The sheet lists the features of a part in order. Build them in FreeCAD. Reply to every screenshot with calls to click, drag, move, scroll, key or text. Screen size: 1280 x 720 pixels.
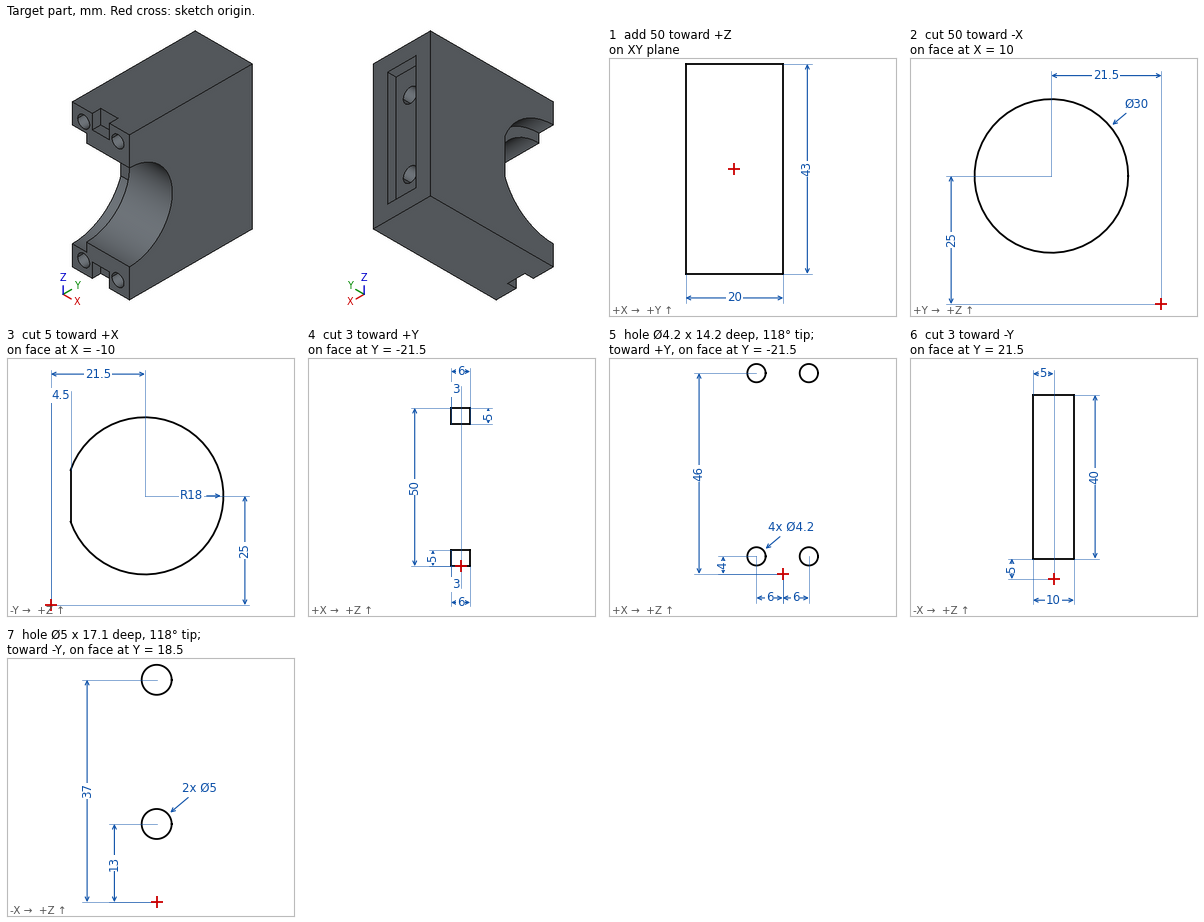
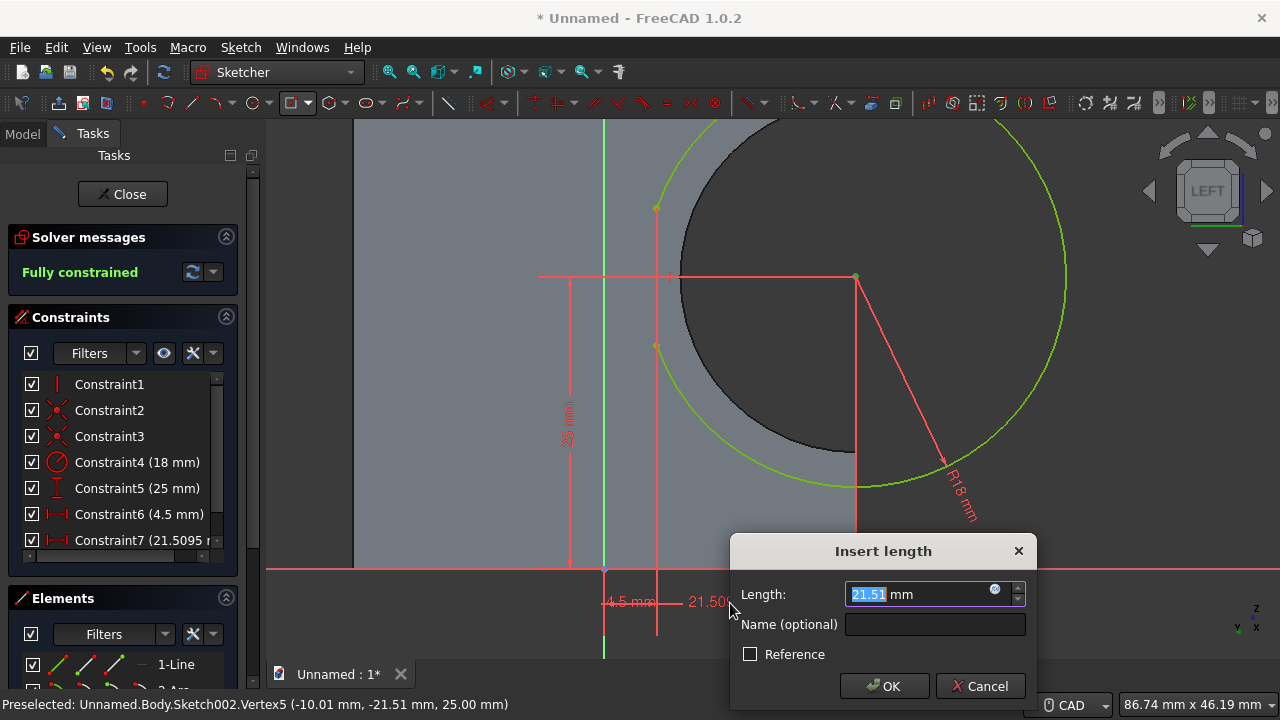
text(21.5)
key(Return)
key(Escape)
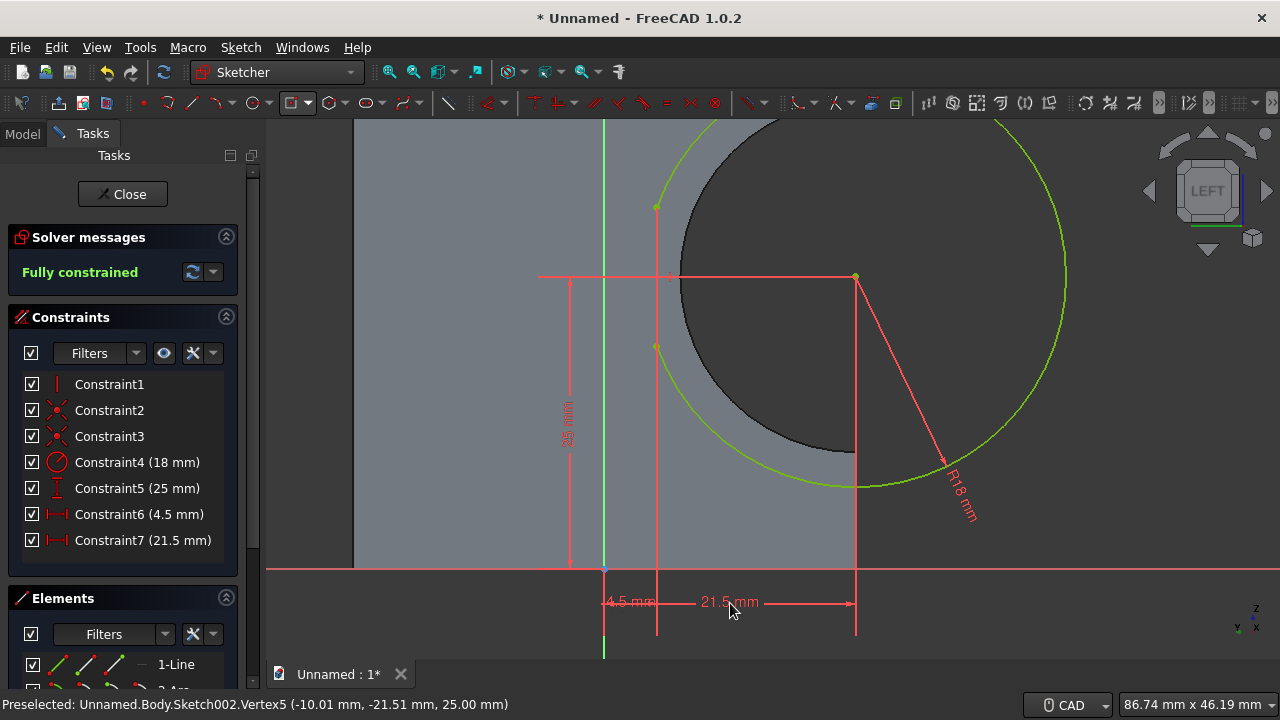
click(123, 194)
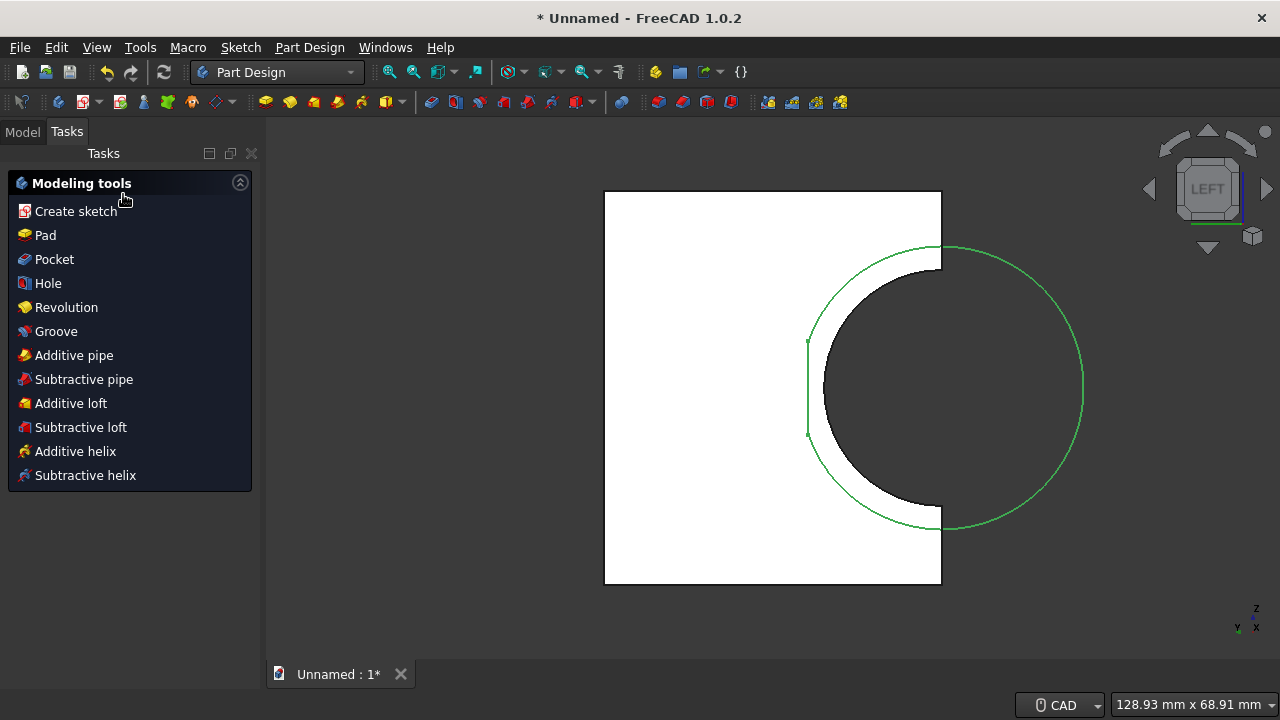
click(432, 102)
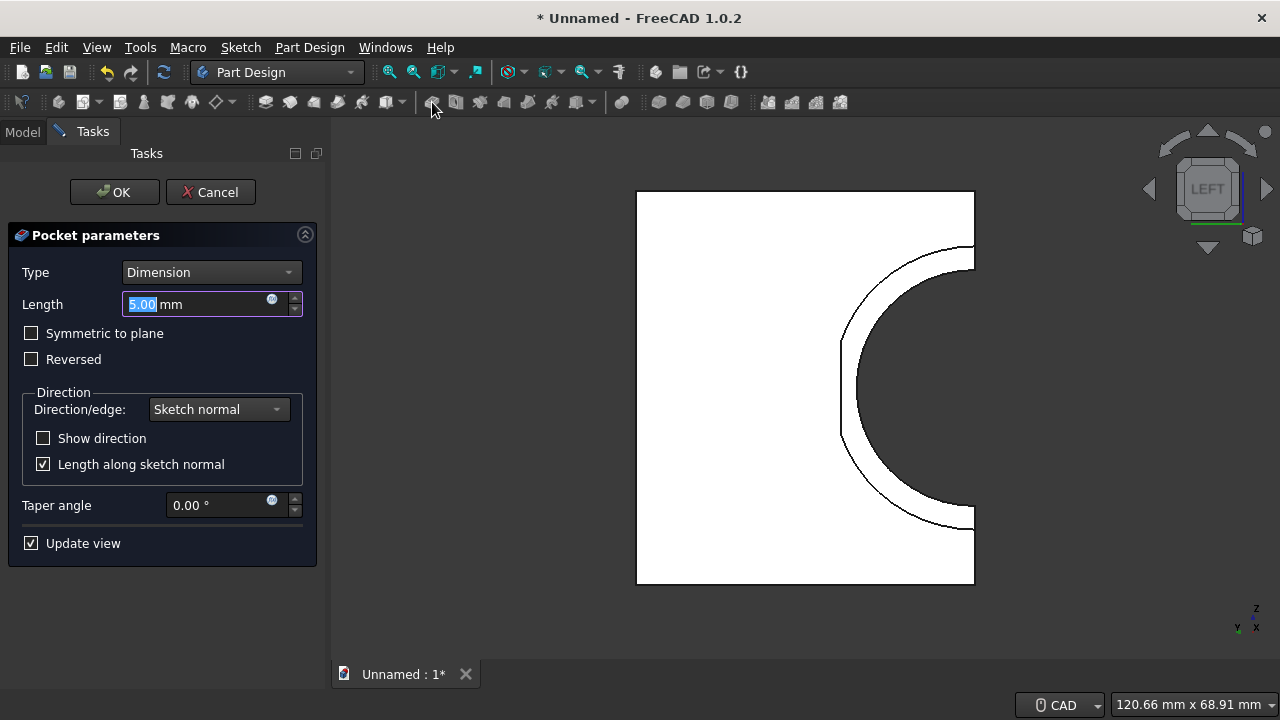
text(5)
key(Tab)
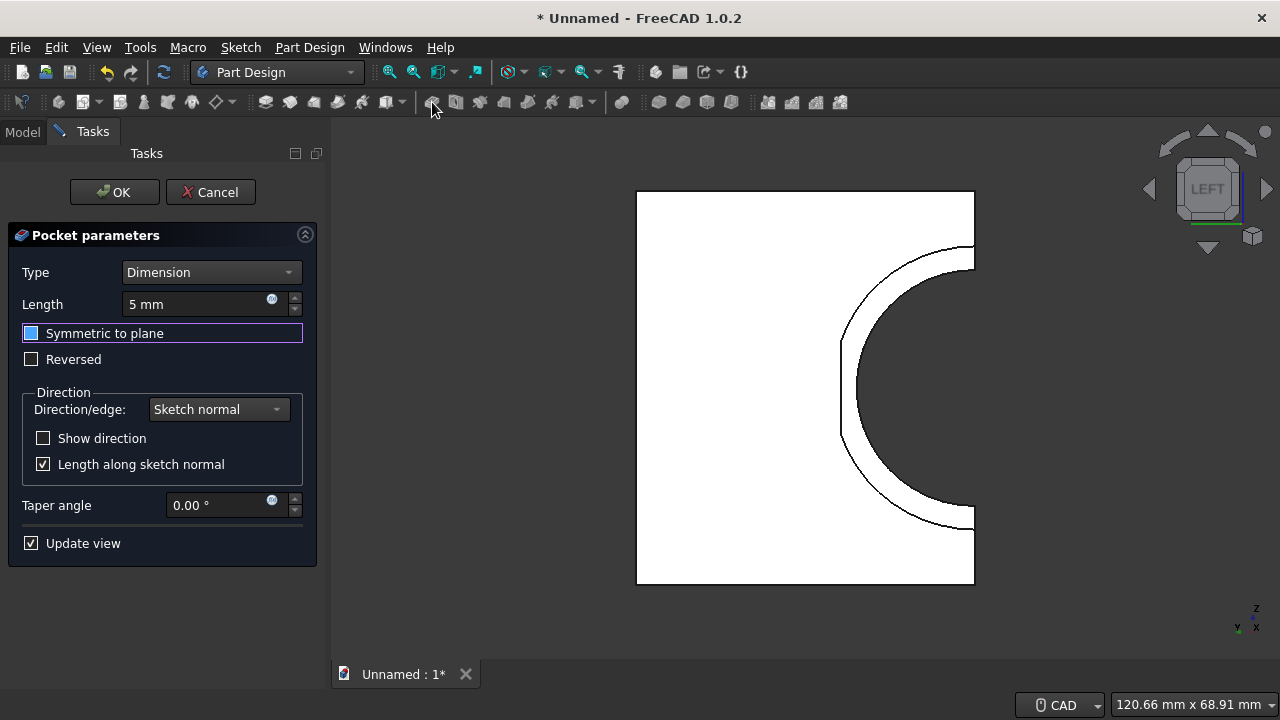
click(115, 192)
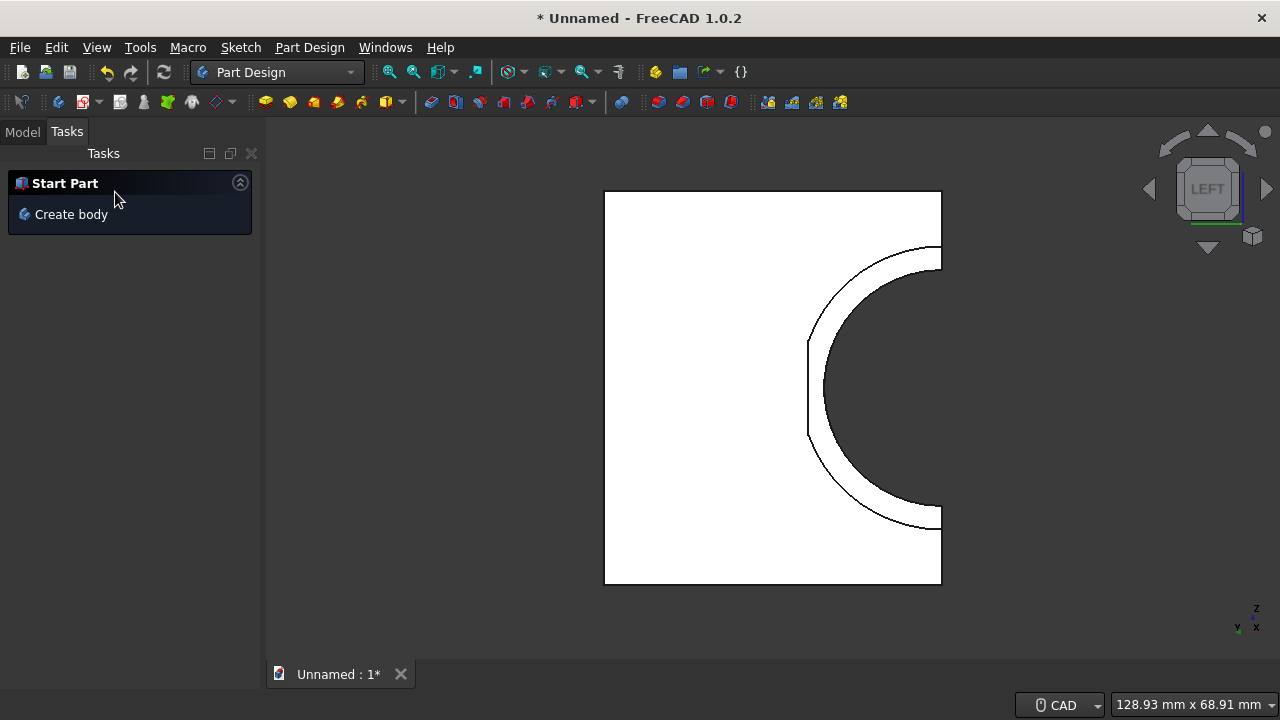
key(0)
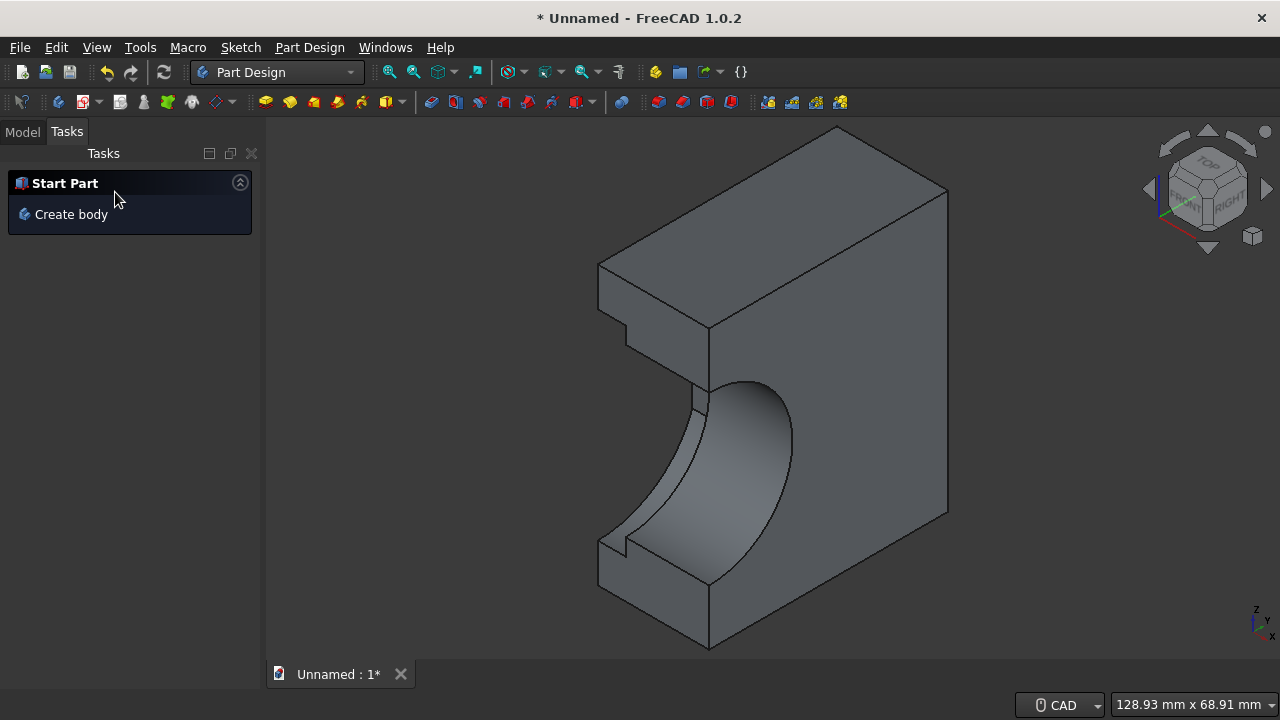
click(669, 337)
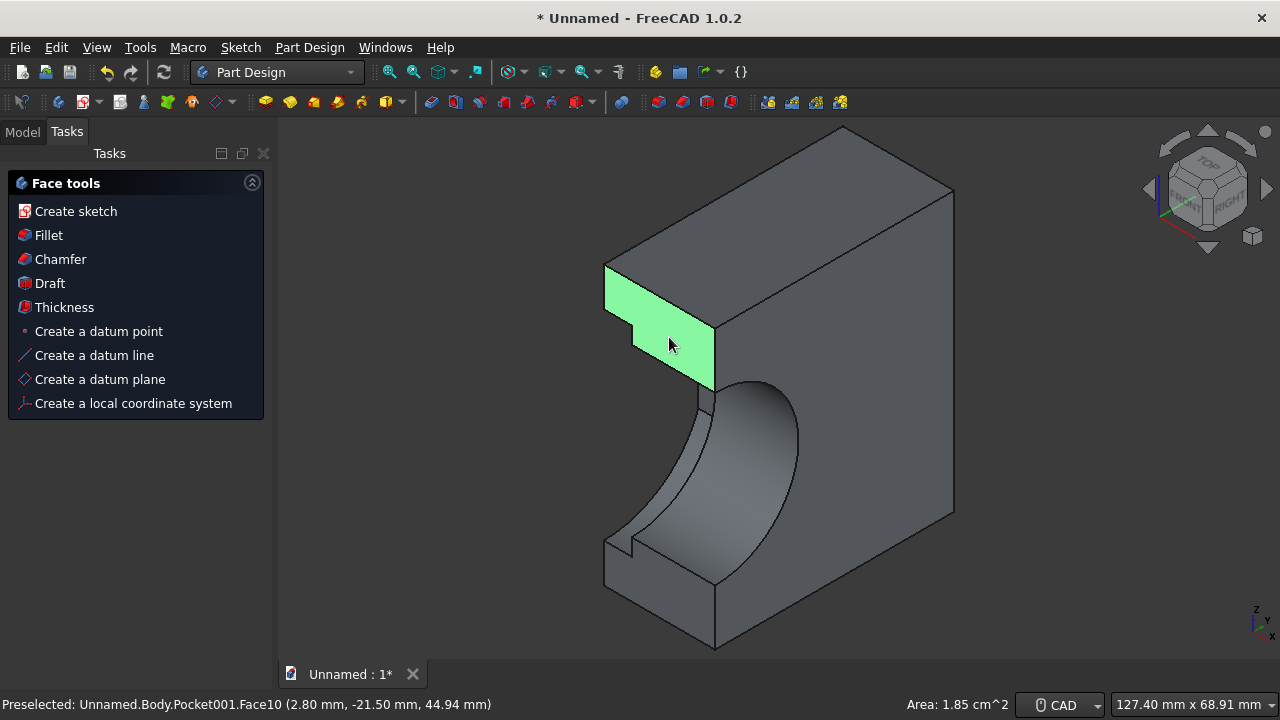
click(84, 102)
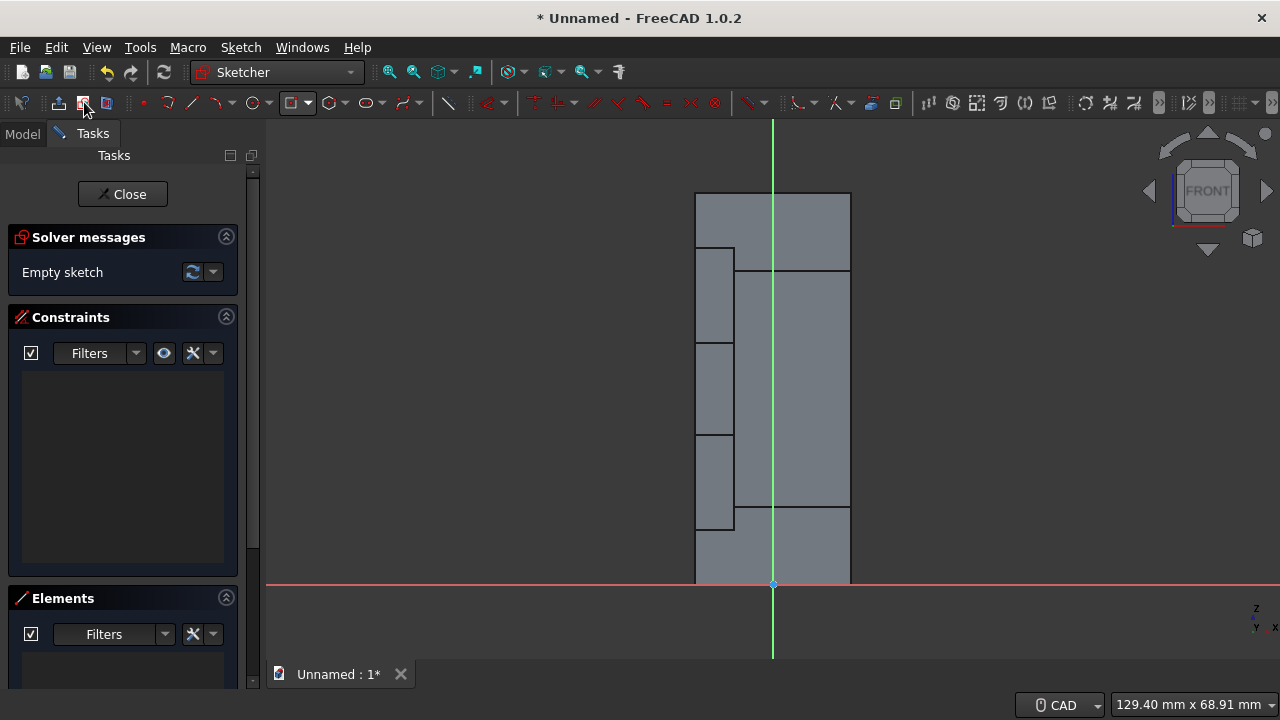
click(310, 104)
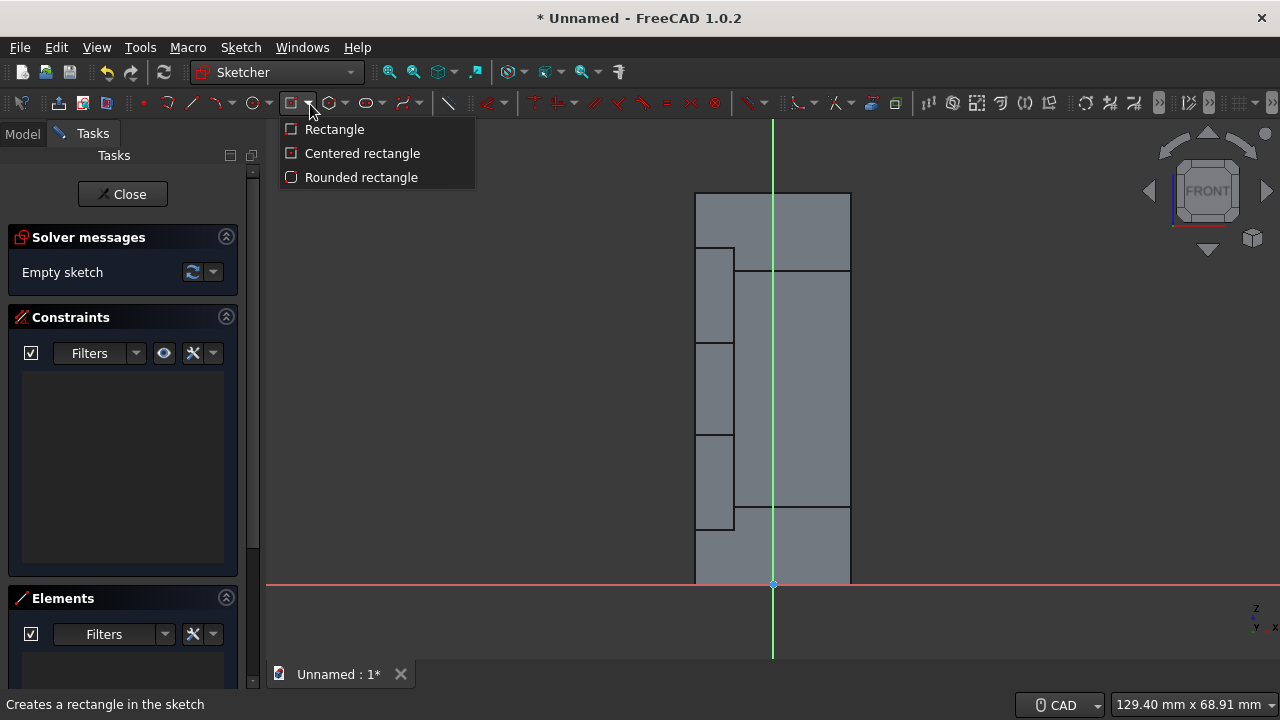
click(378, 129)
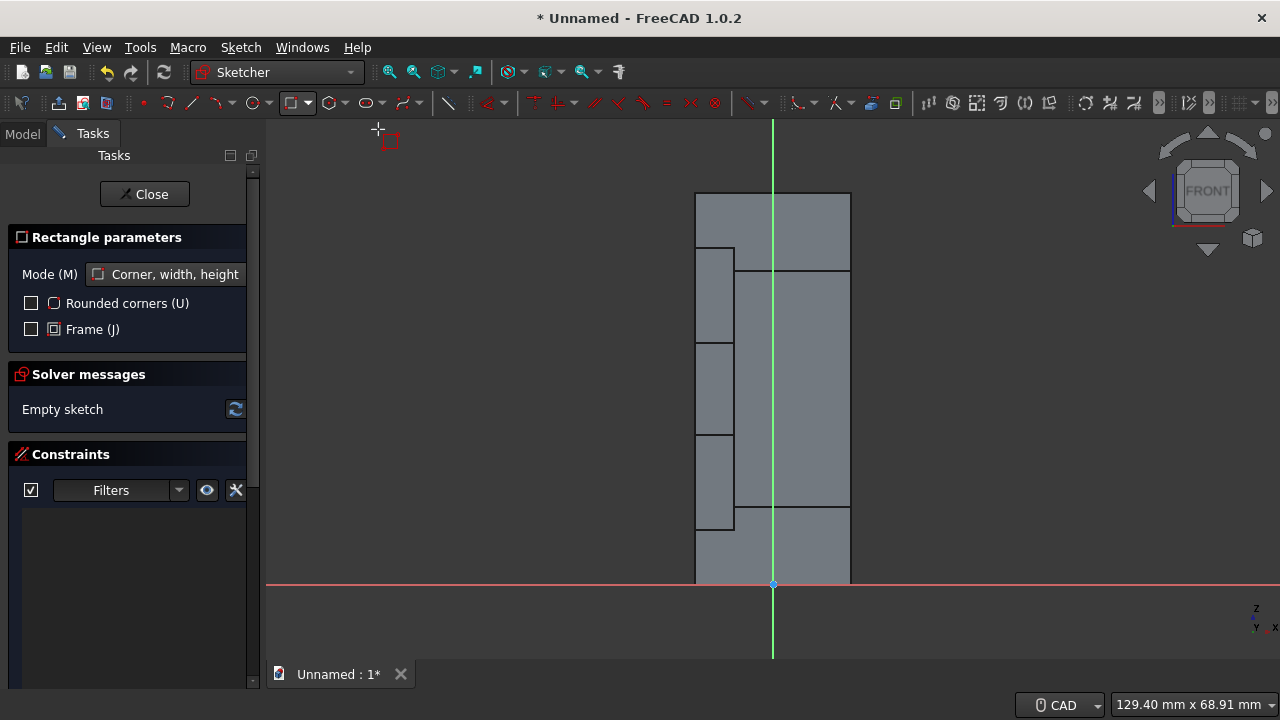
click(749, 546)
click(797, 585)